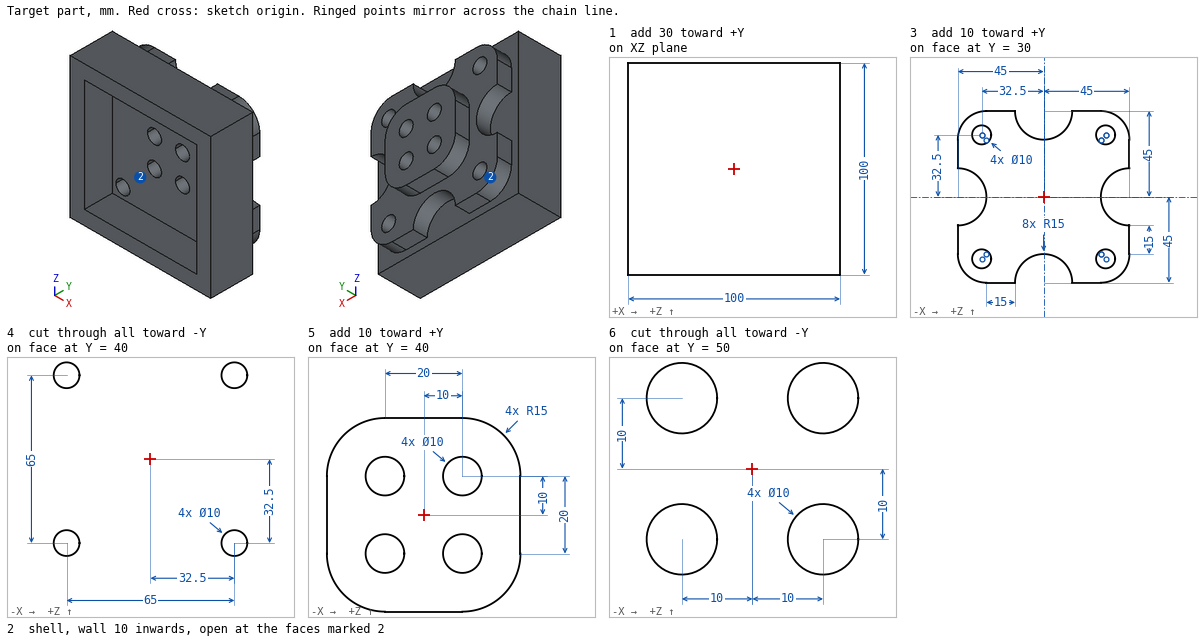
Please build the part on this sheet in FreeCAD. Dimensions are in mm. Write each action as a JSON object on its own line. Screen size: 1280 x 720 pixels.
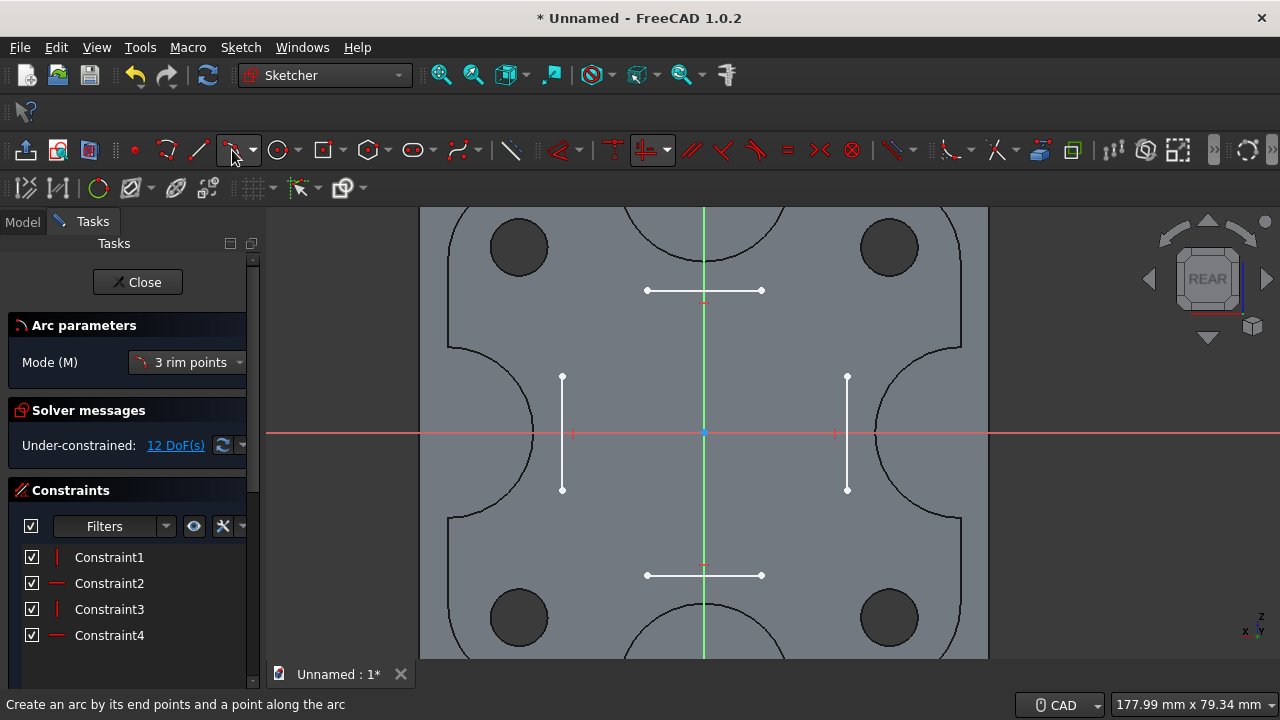
{"action": "left_click", "coordinate": [847, 377]}
{"action": "left_click", "coordinate": [761, 291]}
{"action": "left_click", "coordinate": [822, 315]}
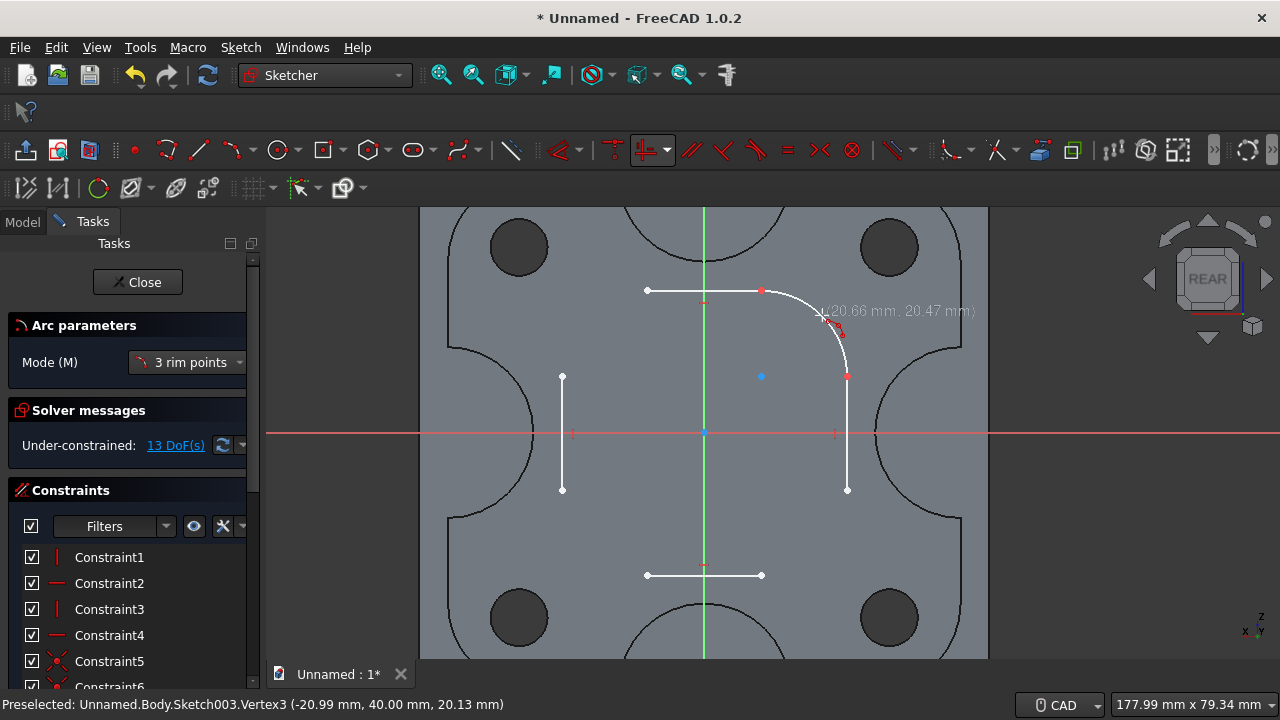
{"action": "left_click", "coordinate": [647, 291]}
{"action": "left_click", "coordinate": [562, 377]}
{"action": "left_click", "coordinate": [587, 315]}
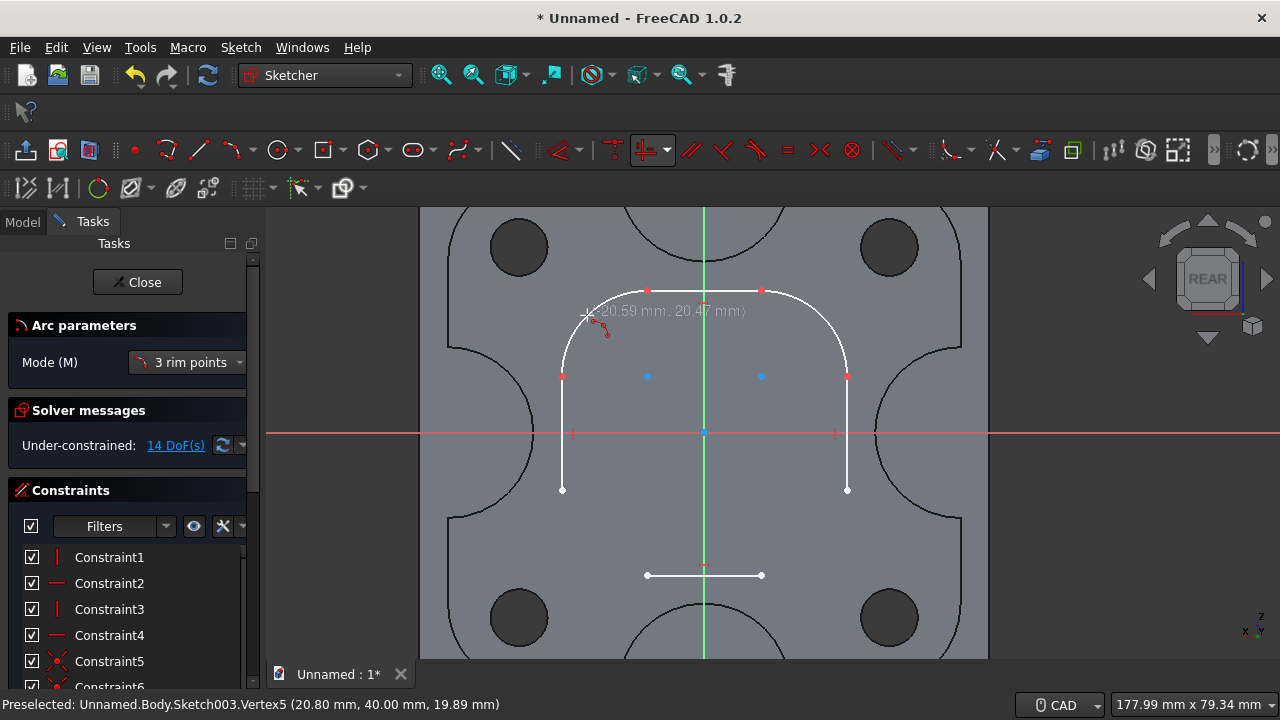
{"action": "left_click", "coordinate": [562, 491]}
{"action": "left_click", "coordinate": [647, 576]}
{"action": "left_click", "coordinate": [587, 550]}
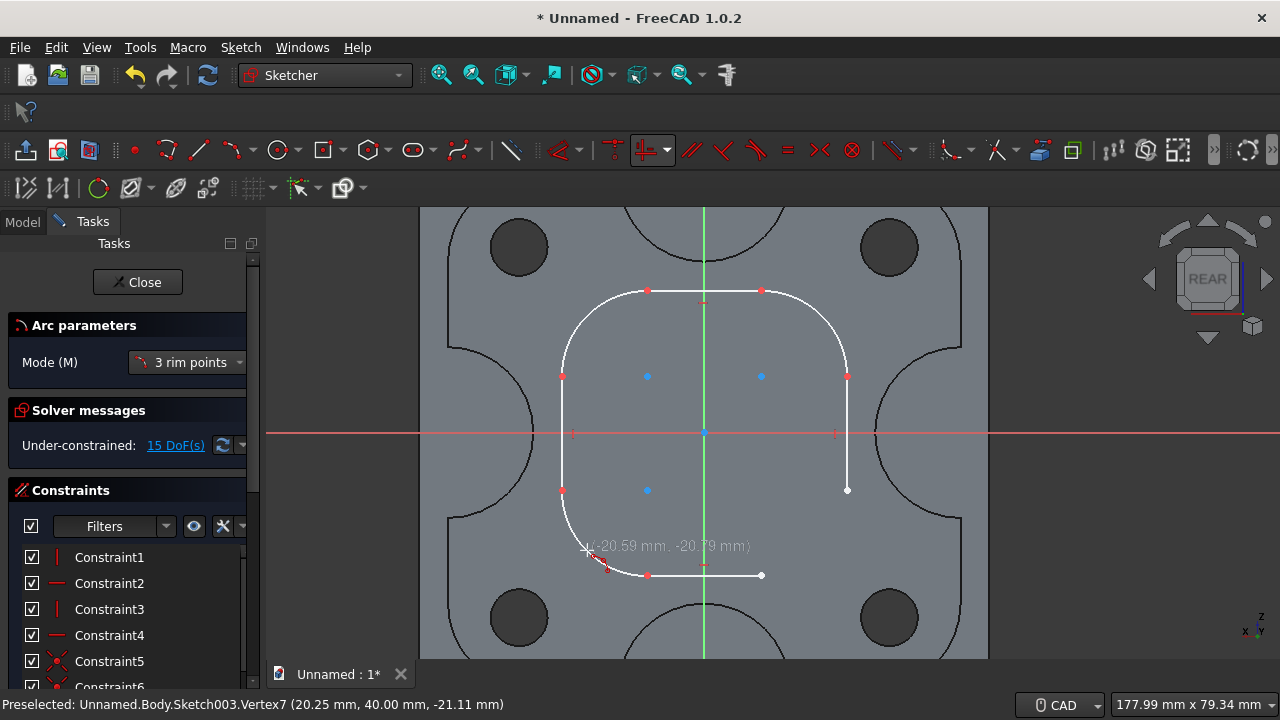
{"action": "left_click", "coordinate": [761, 576]}
{"action": "left_click", "coordinate": [847, 491]}
{"action": "left_click", "coordinate": [822, 550]}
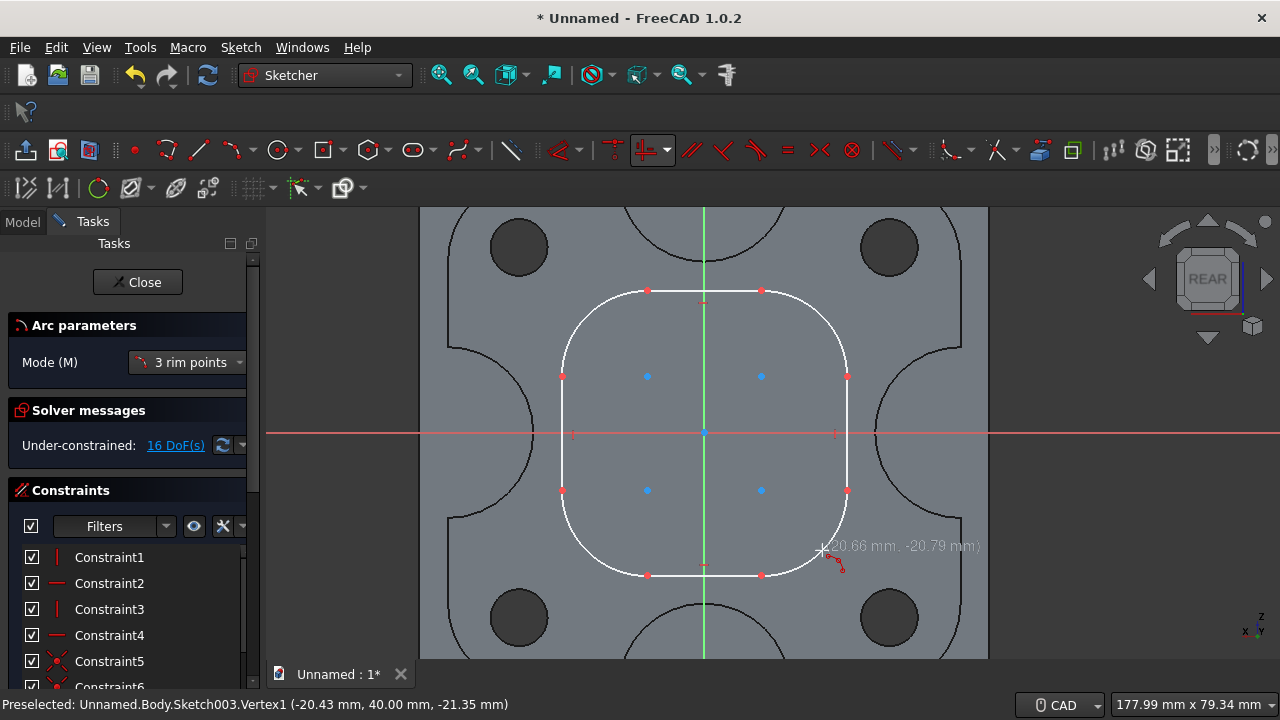
{"action": "left_click", "coordinate": [278, 150]}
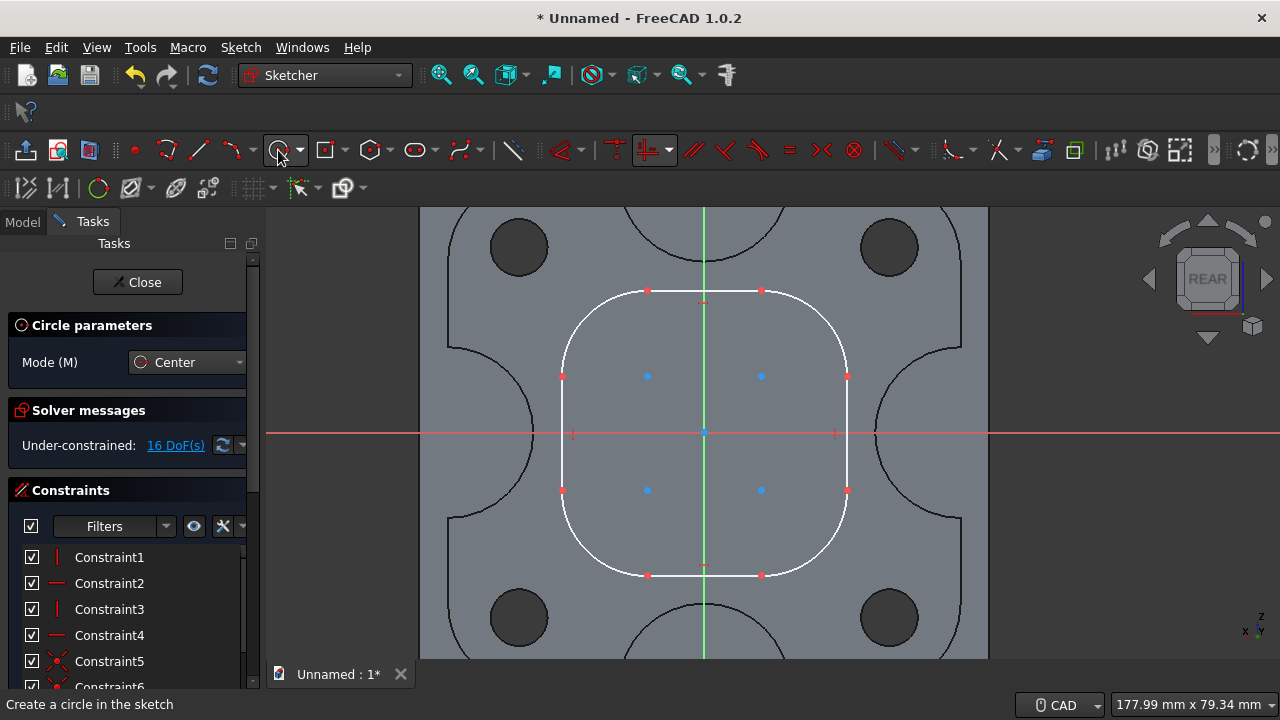
{"action": "left_click", "coordinate": [761, 376]}
{"action": "left_click", "coordinate": [781, 355]}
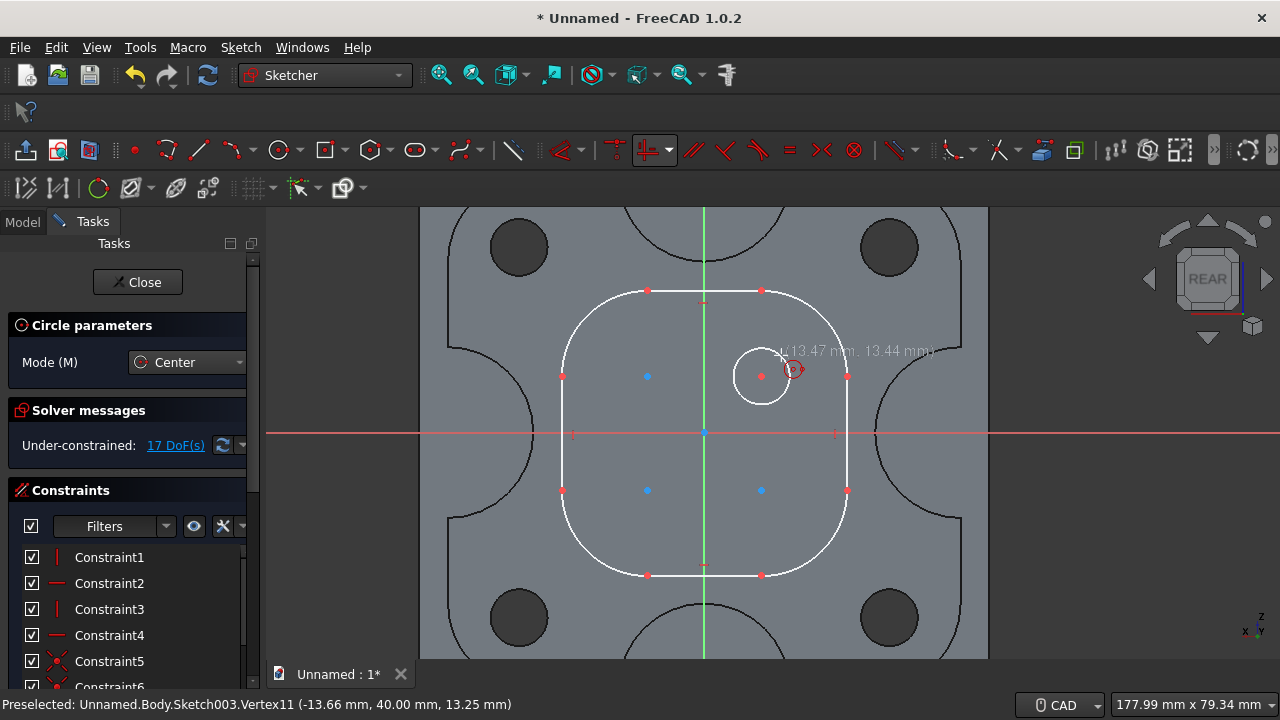
{"action": "left_click", "coordinate": [647, 376]}
{"action": "left_click", "coordinate": [667, 355]}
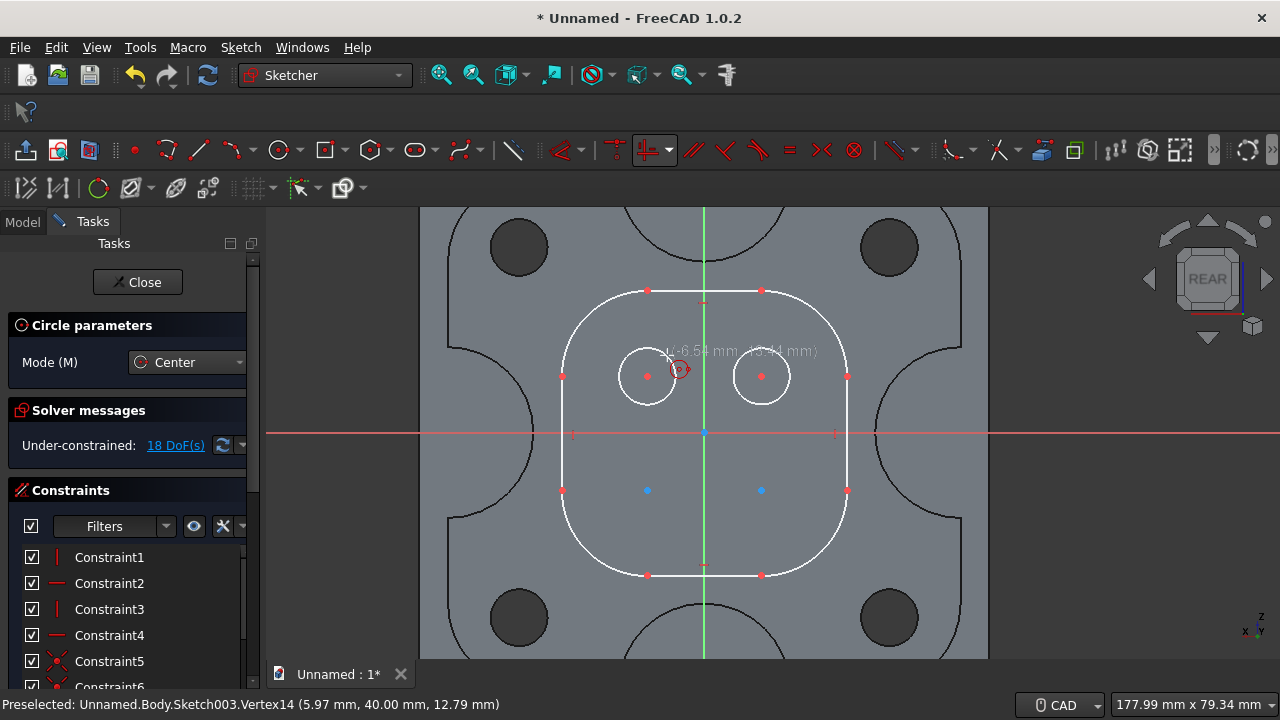
{"action": "left_click", "coordinate": [761, 490]}
{"action": "left_click", "coordinate": [781, 469]}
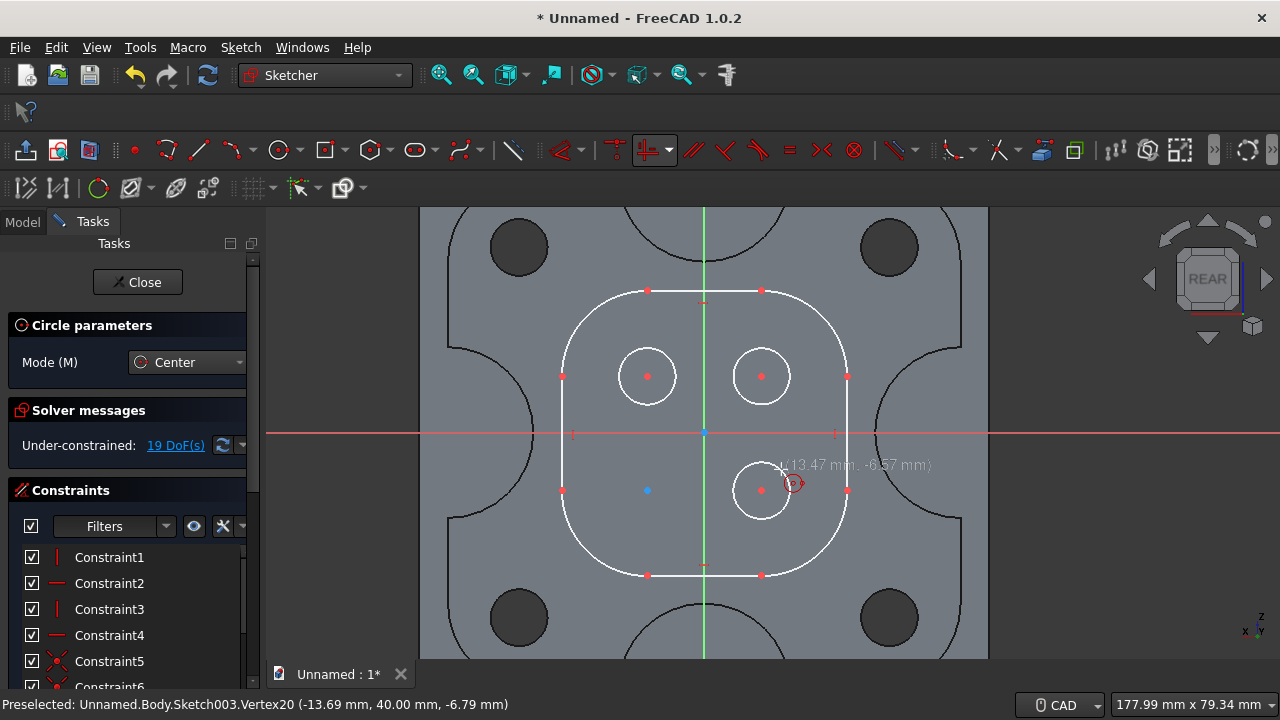
{"action": "left_click", "coordinate": [647, 490]}
{"action": "left_click", "coordinate": [667, 469]}
{"action": "key", "text": "Escape"}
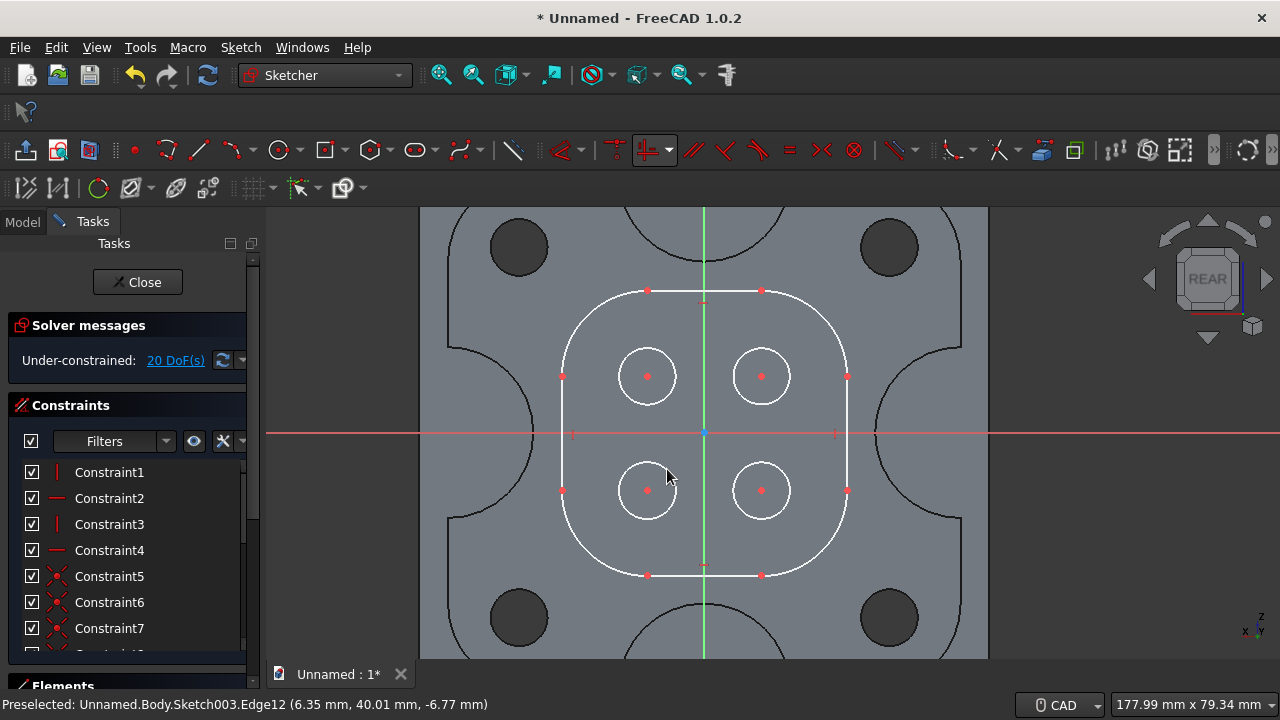
{"action": "left_click", "coordinate": [847, 457]}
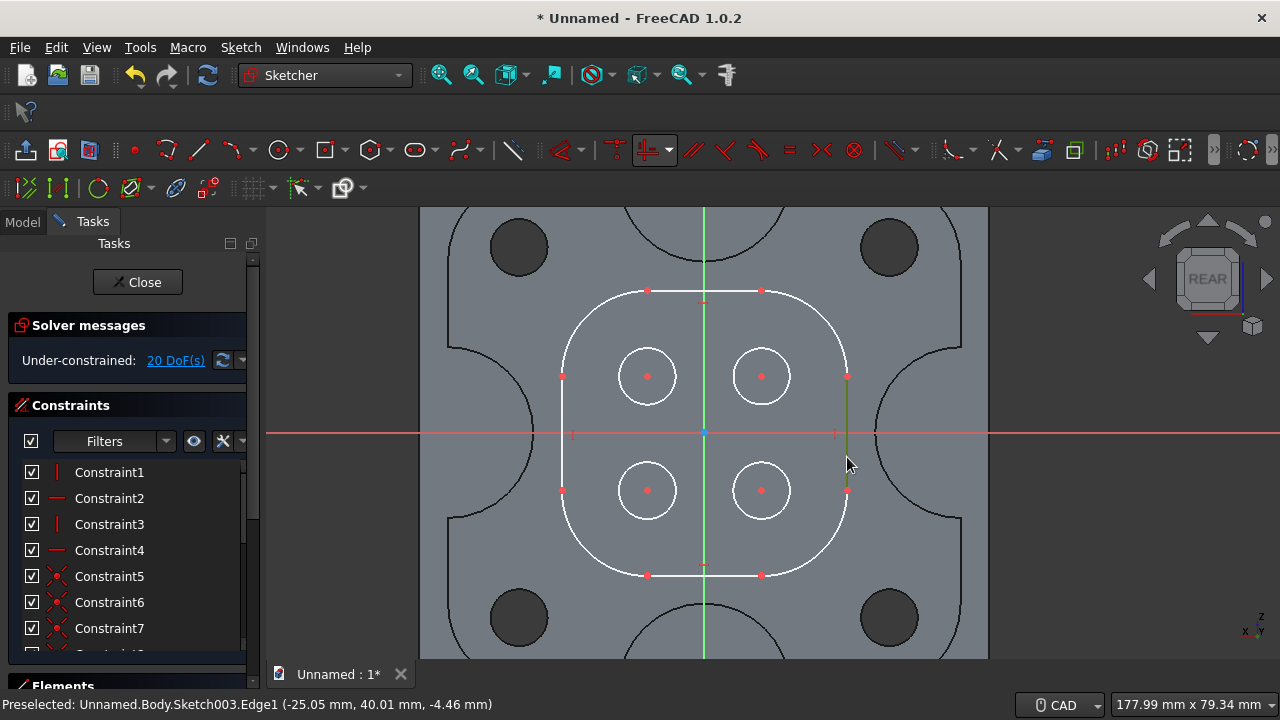
{"action": "left_click", "coordinate": [838, 338]}